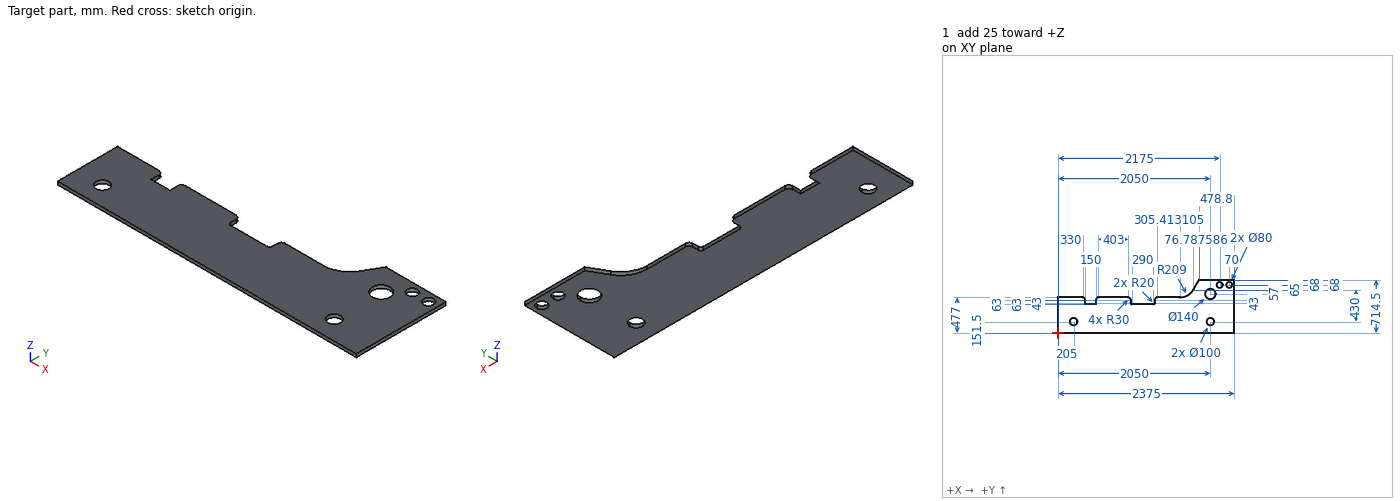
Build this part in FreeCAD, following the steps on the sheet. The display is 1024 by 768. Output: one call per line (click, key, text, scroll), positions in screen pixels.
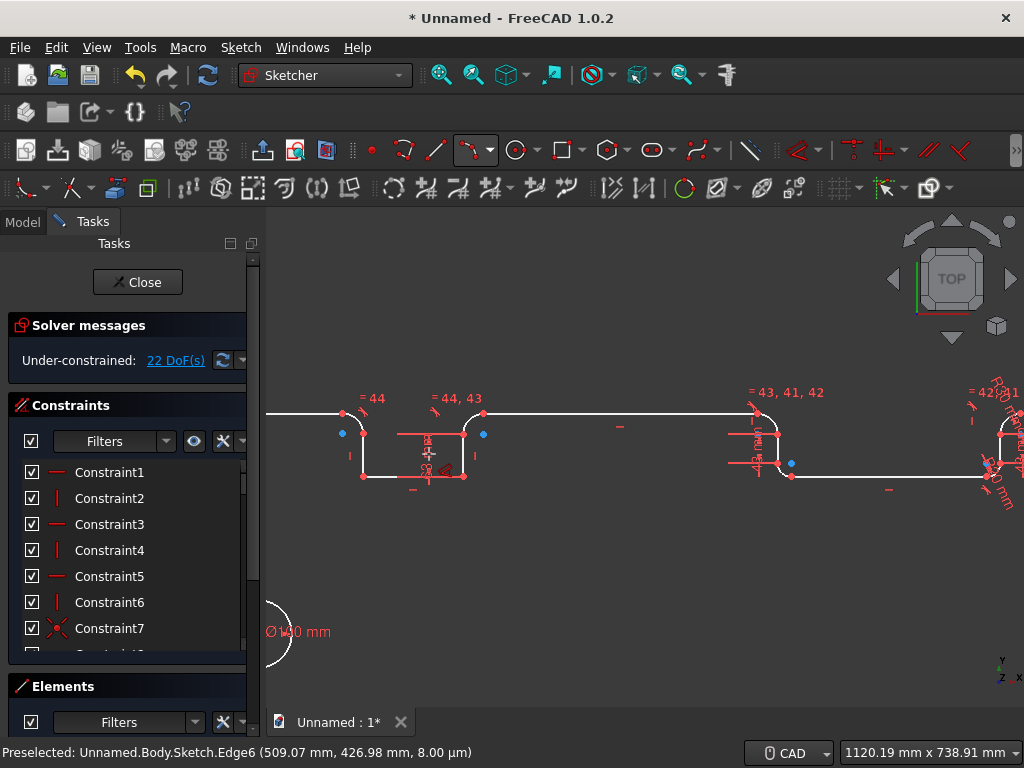
click(363, 464)
click(329, 455)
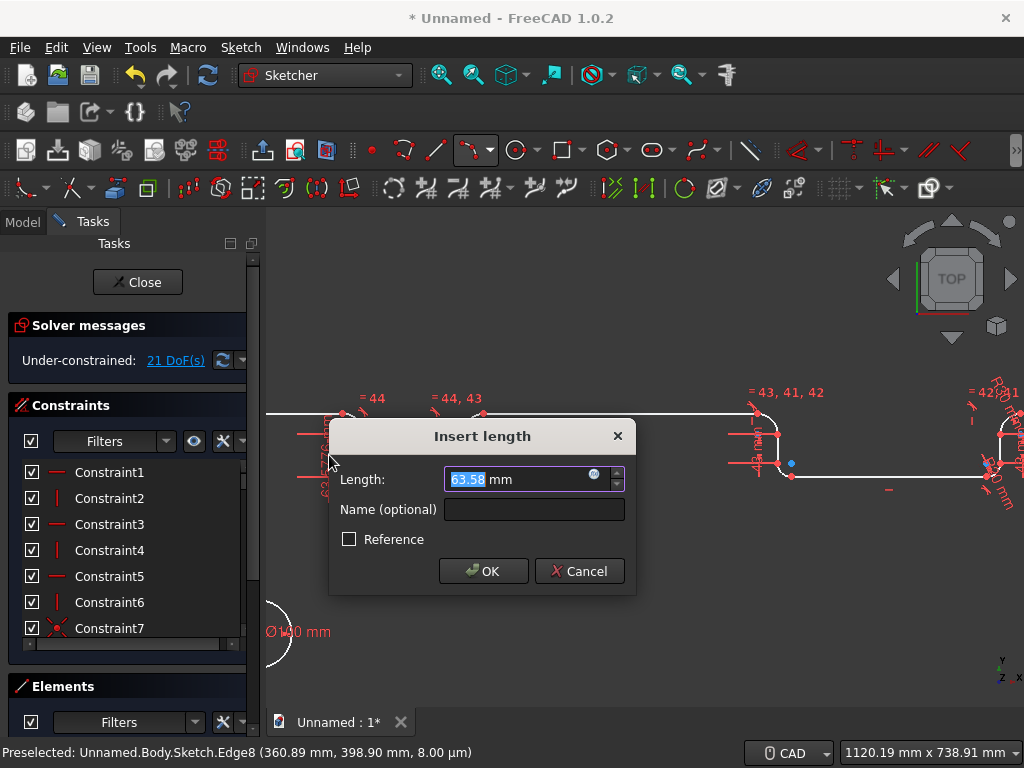
text(63)
key(Return)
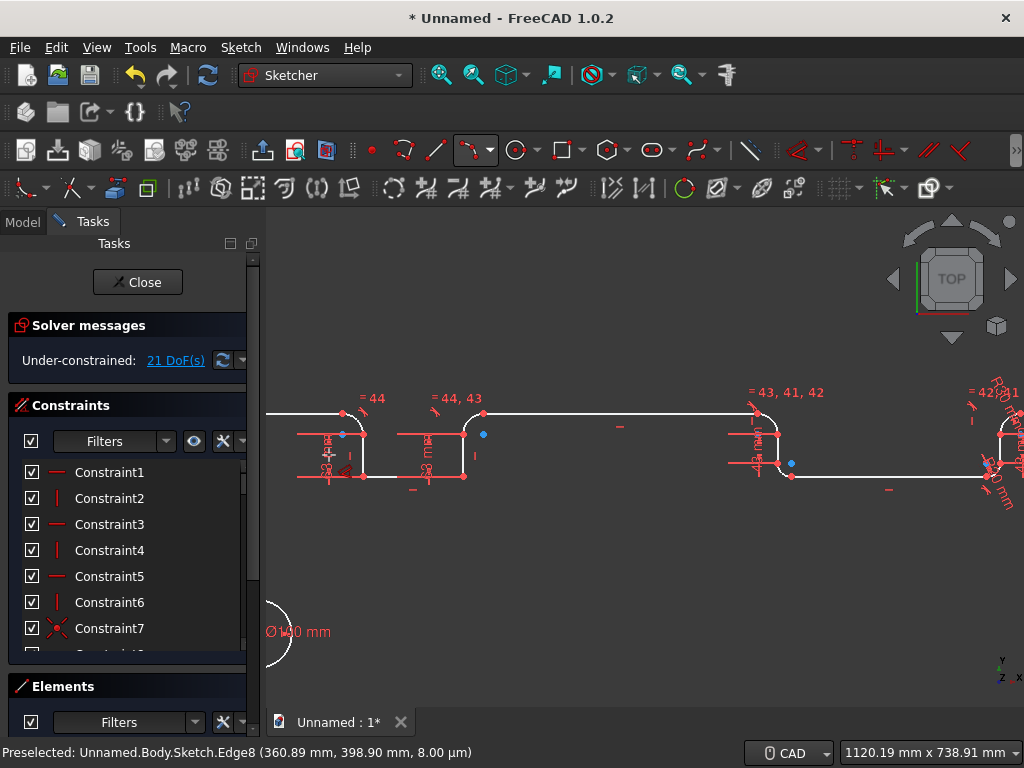
click(850, 477)
click(841, 443)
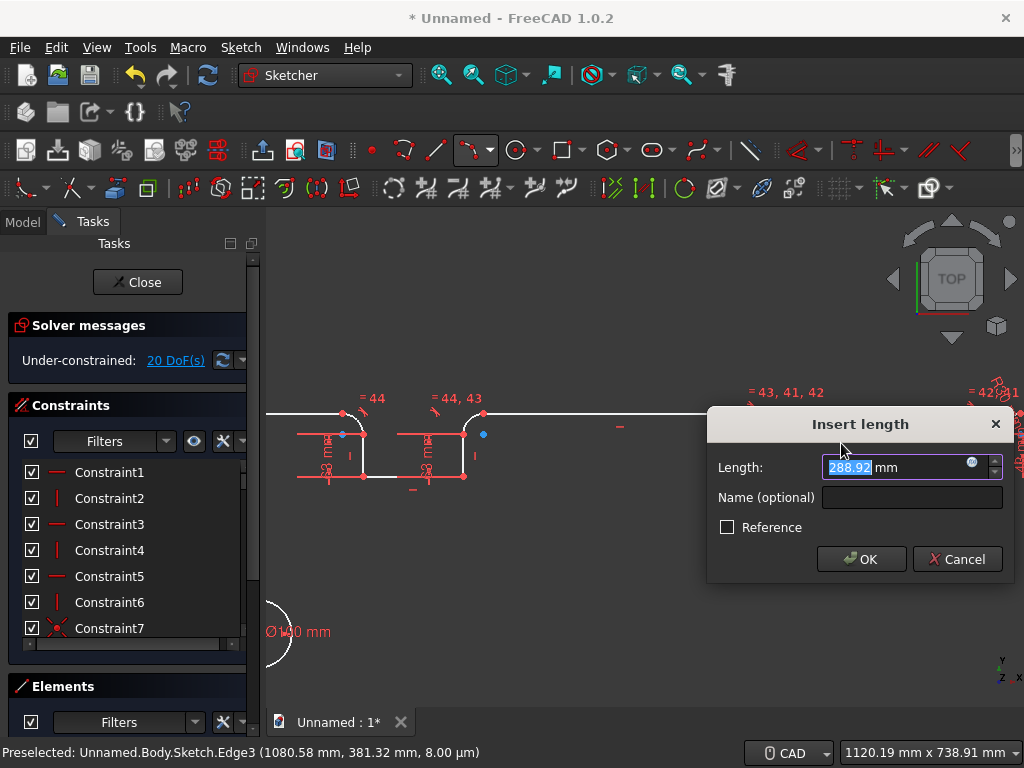
text(290)
key(Return)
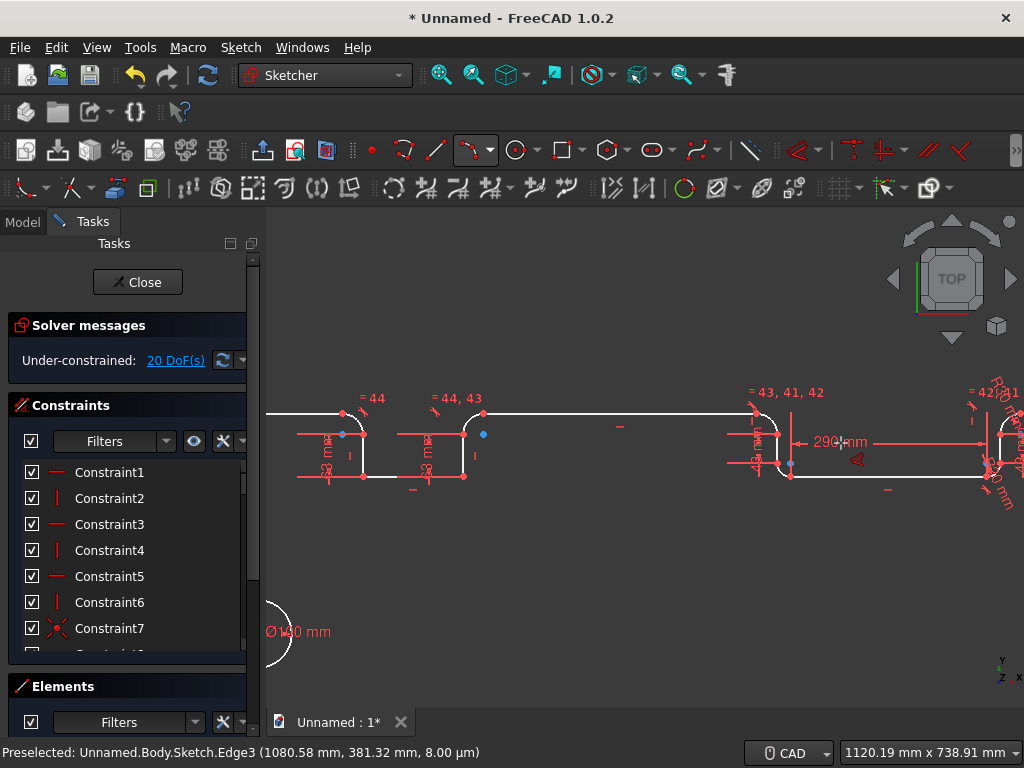
click(675, 414)
click(620, 380)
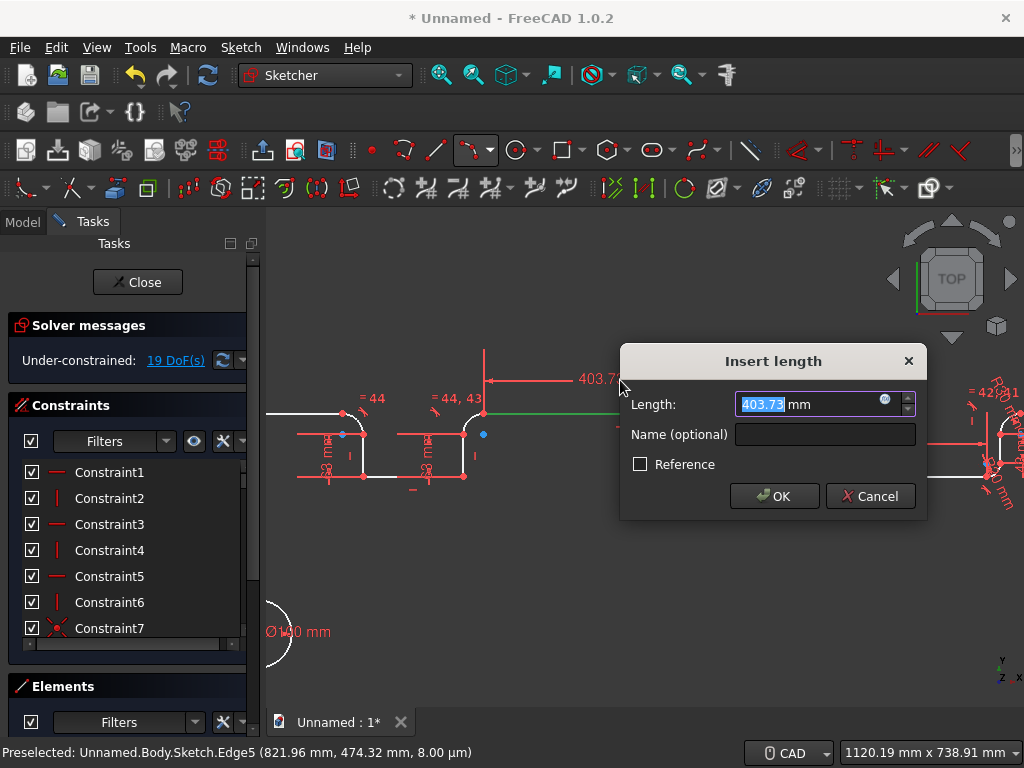
text(403)
key(Return)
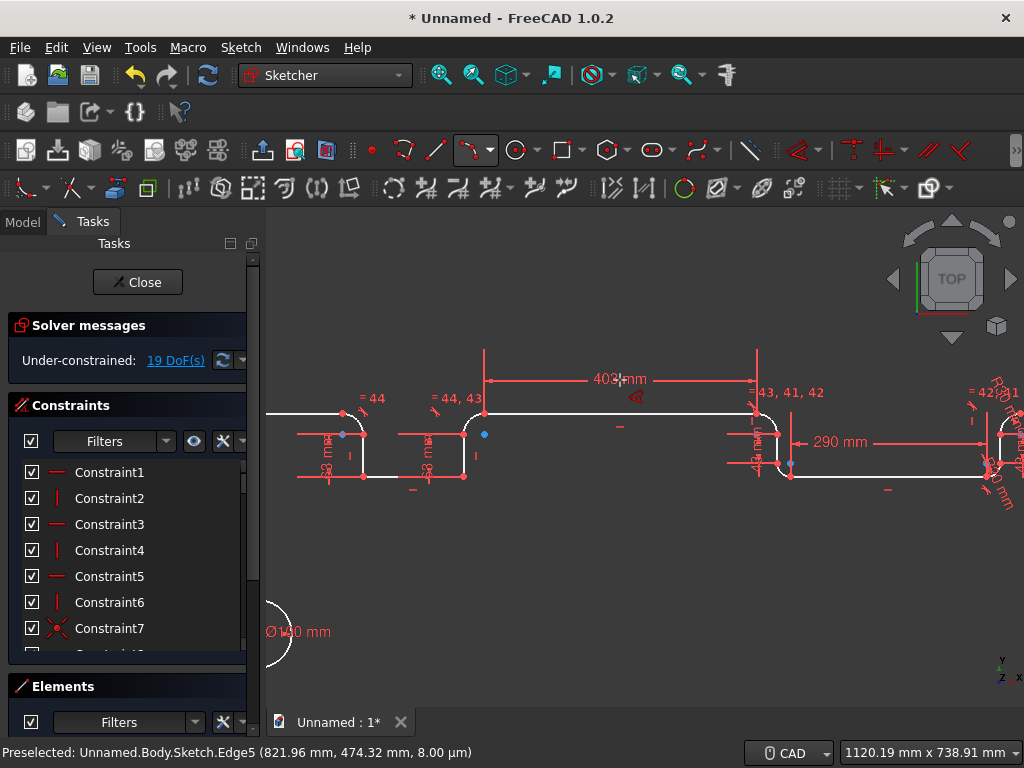
click(434, 477)
click(413, 511)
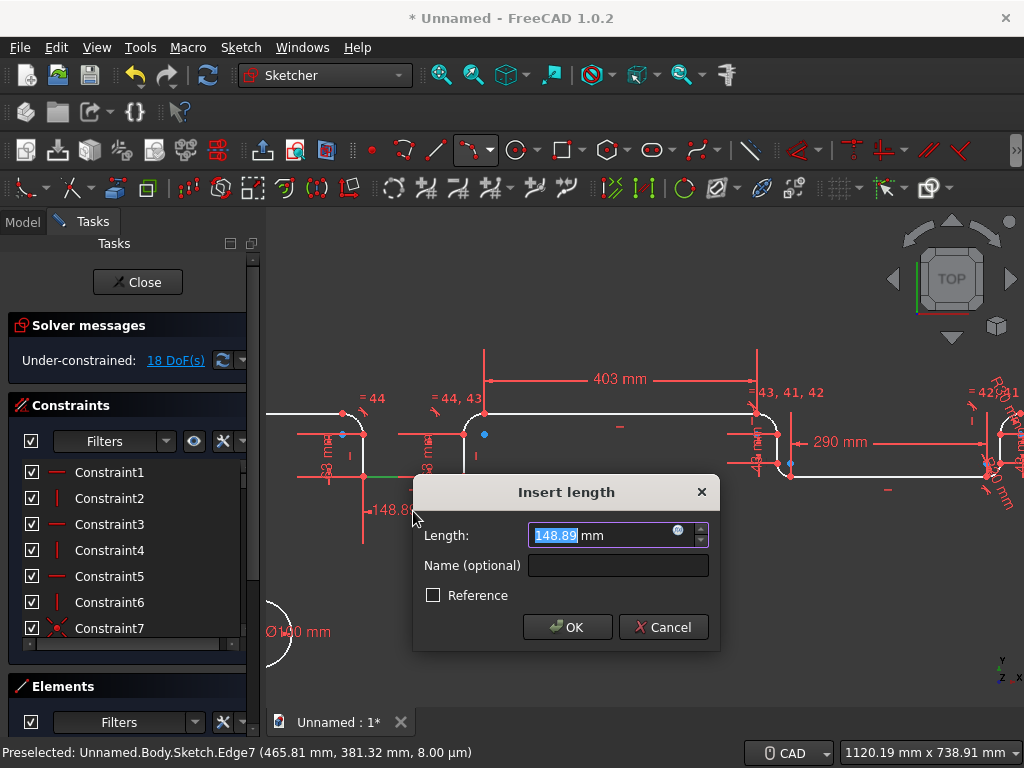
text(150)
key(Return)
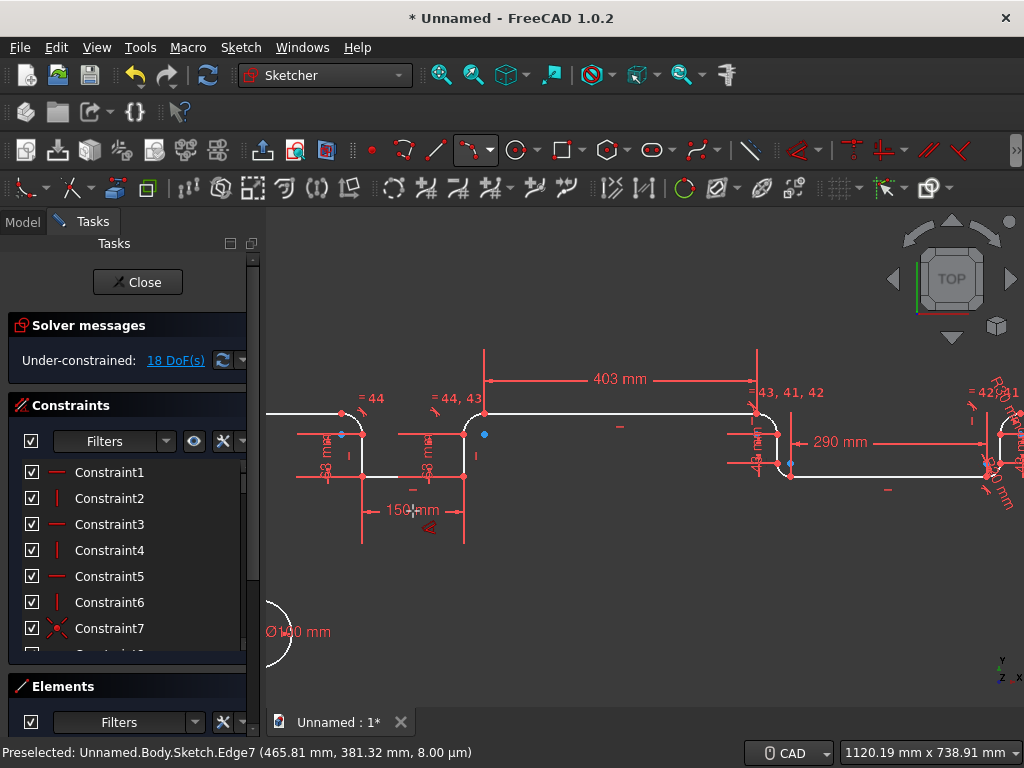
click(297, 414)
click(318, 380)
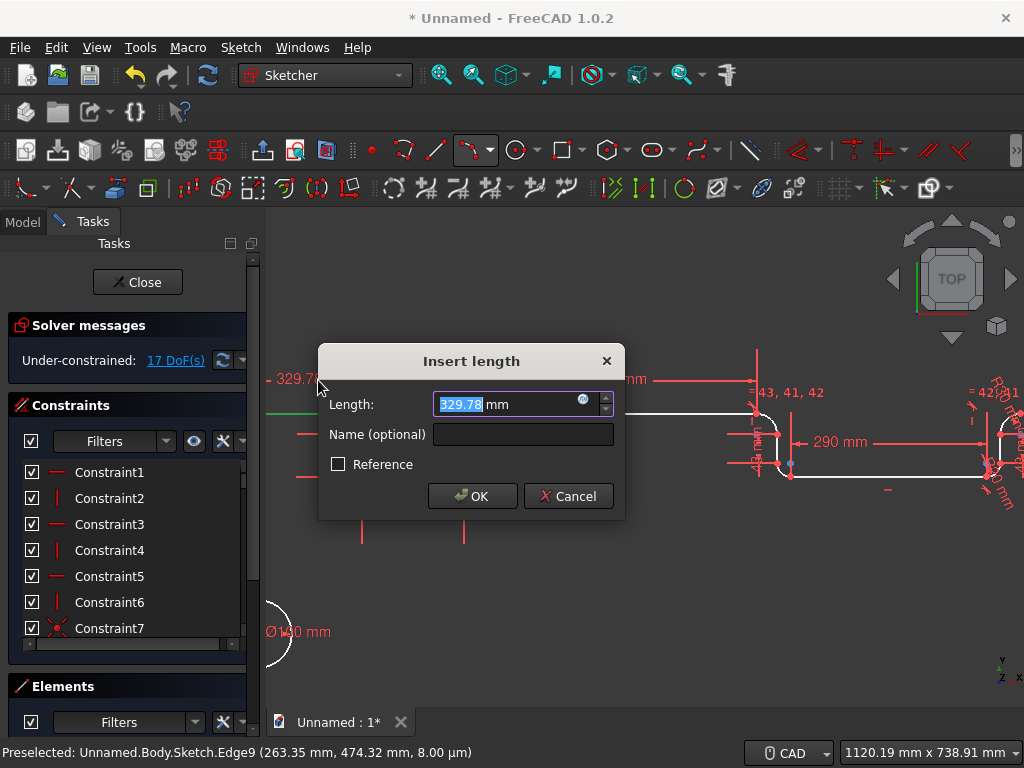
text(330)
key(Return)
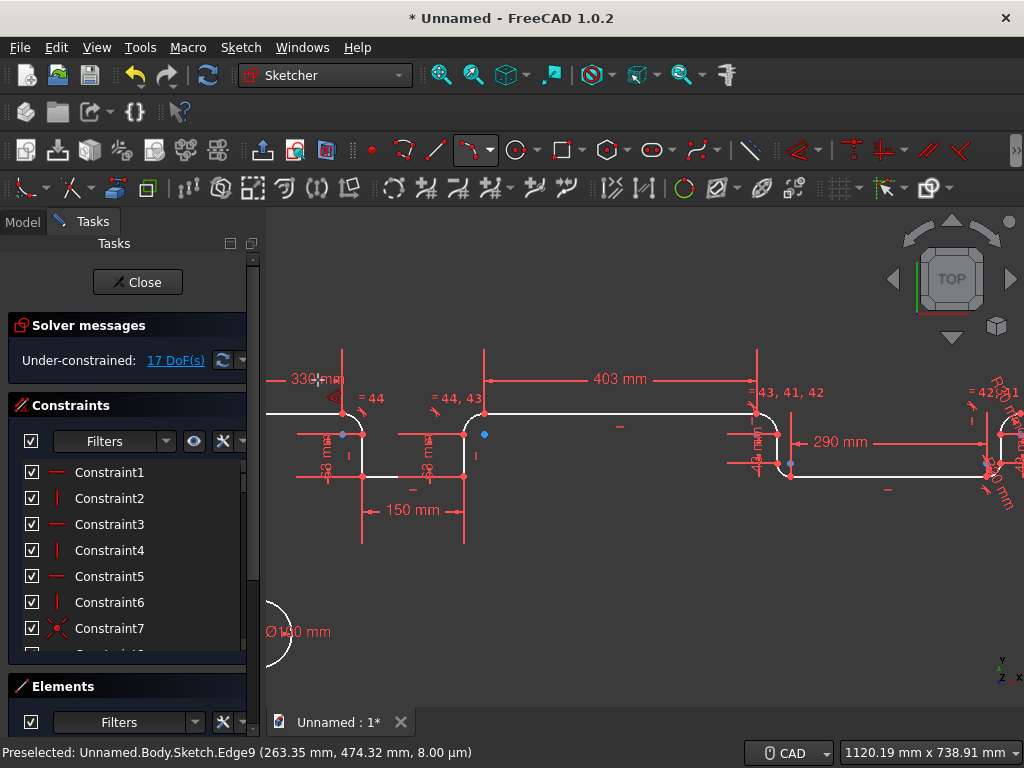
scroll(463, 445, down, 7)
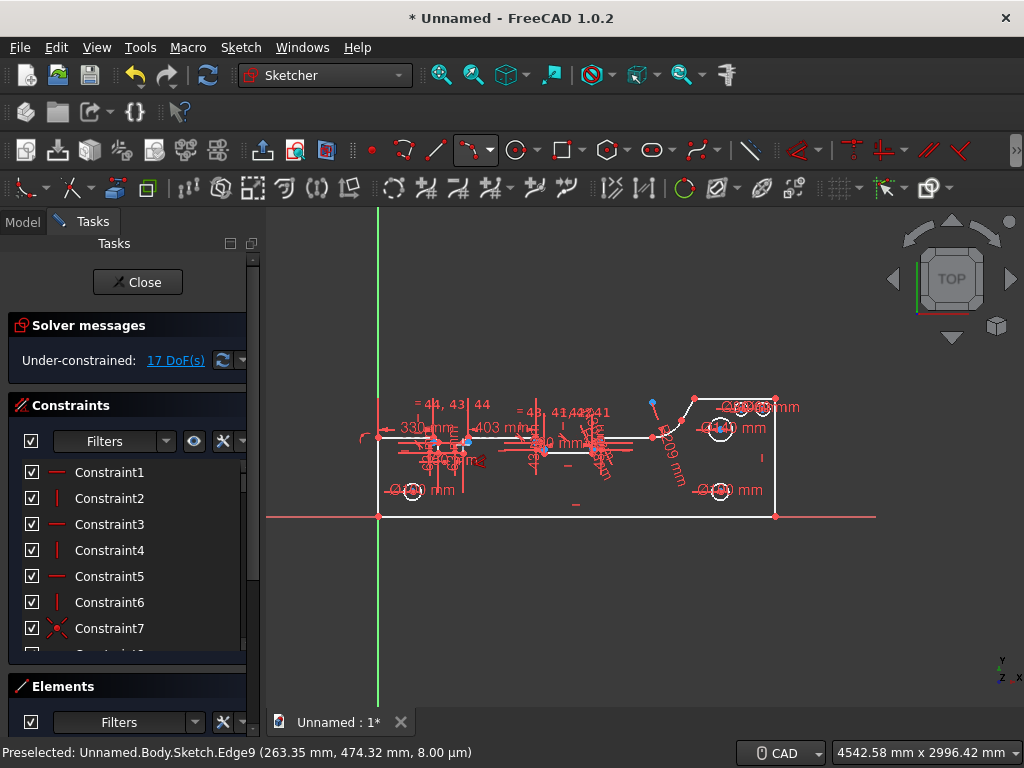
click(378, 461)
click(344, 477)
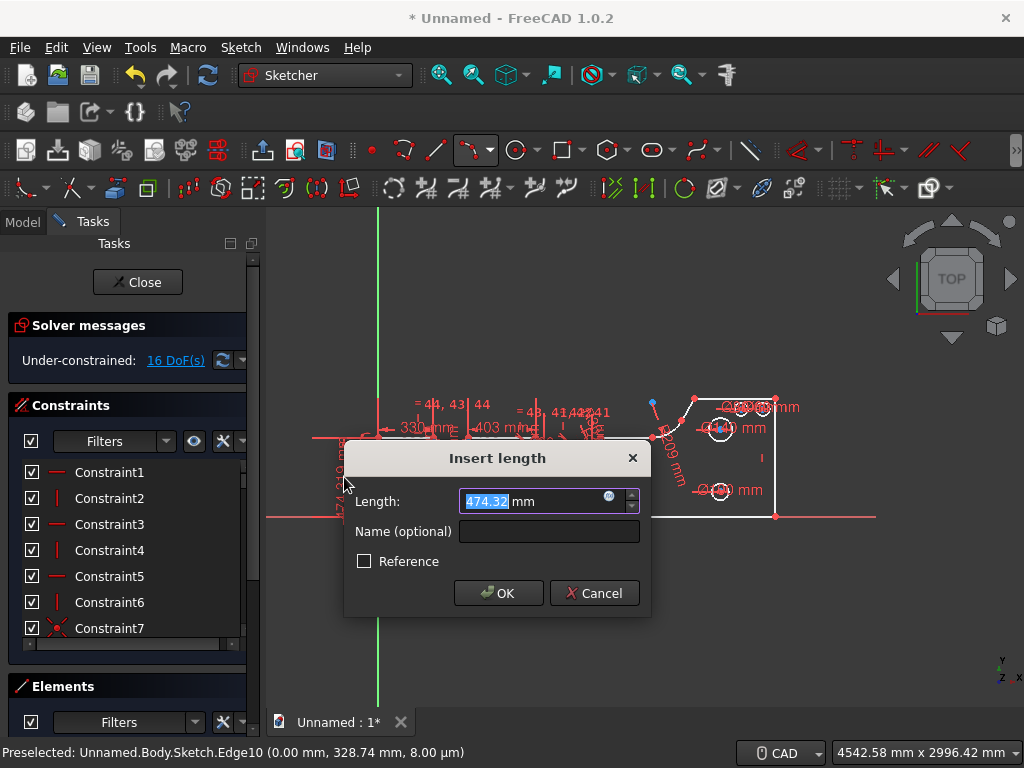
text(477)
key(Return)